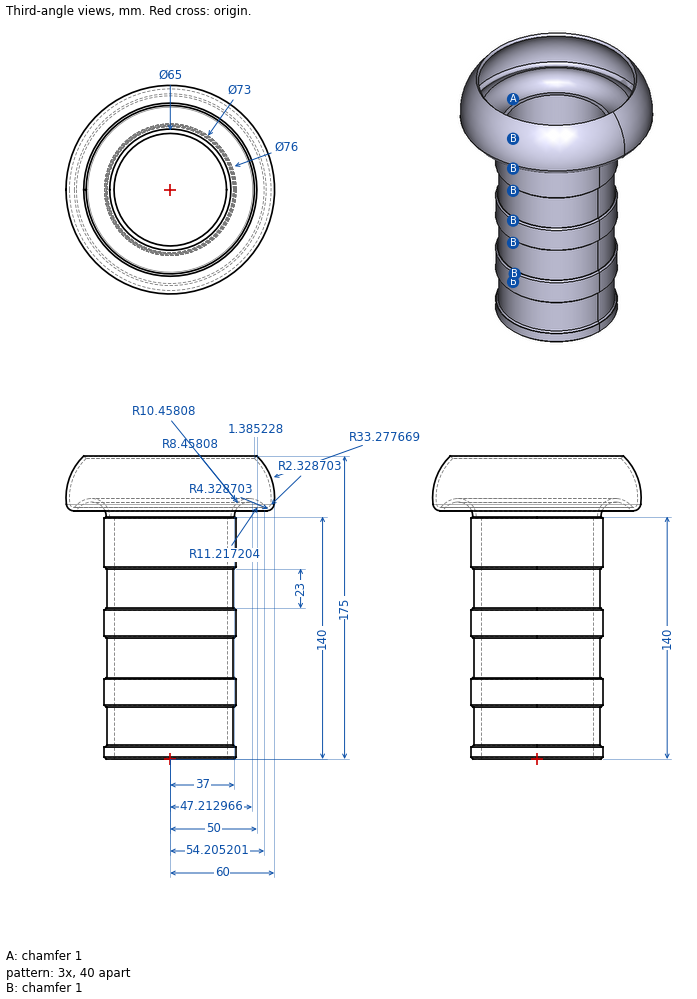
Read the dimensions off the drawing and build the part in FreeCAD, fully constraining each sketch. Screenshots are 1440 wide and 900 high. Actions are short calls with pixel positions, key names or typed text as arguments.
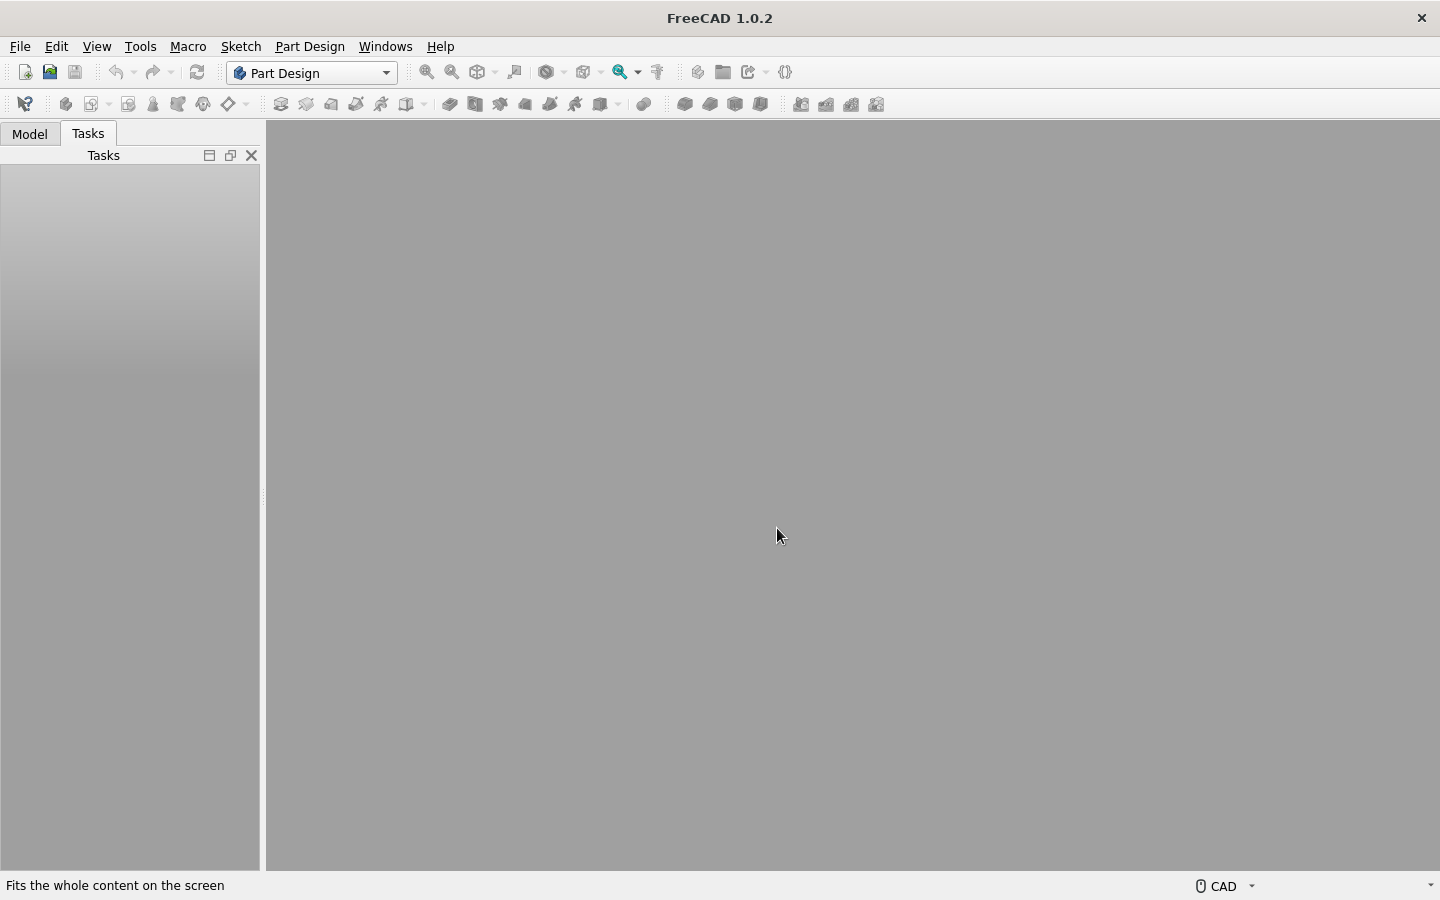
key(ctrl+n)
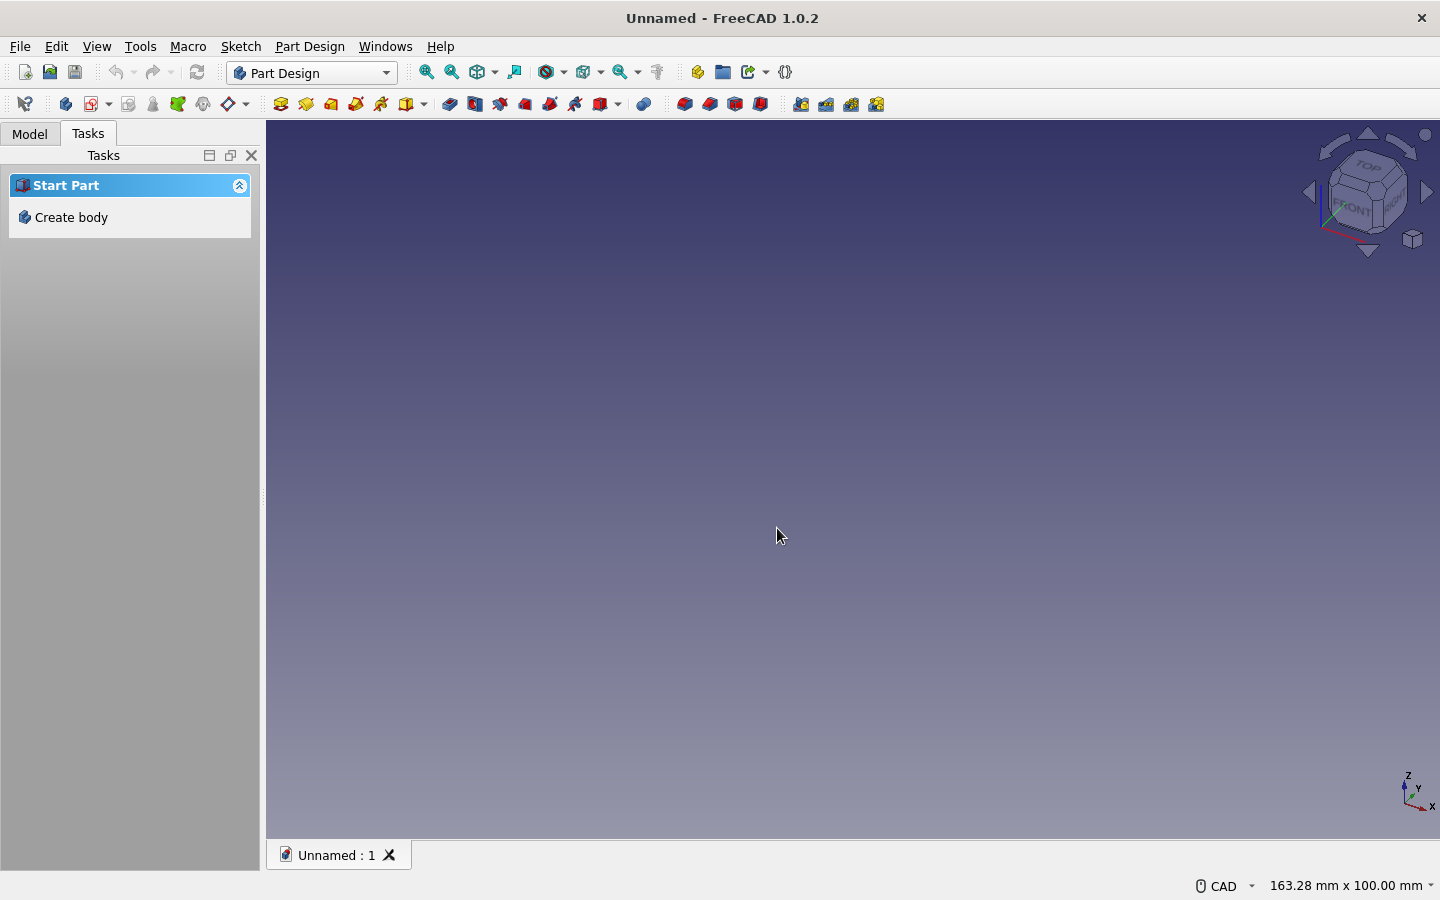
click(90, 104)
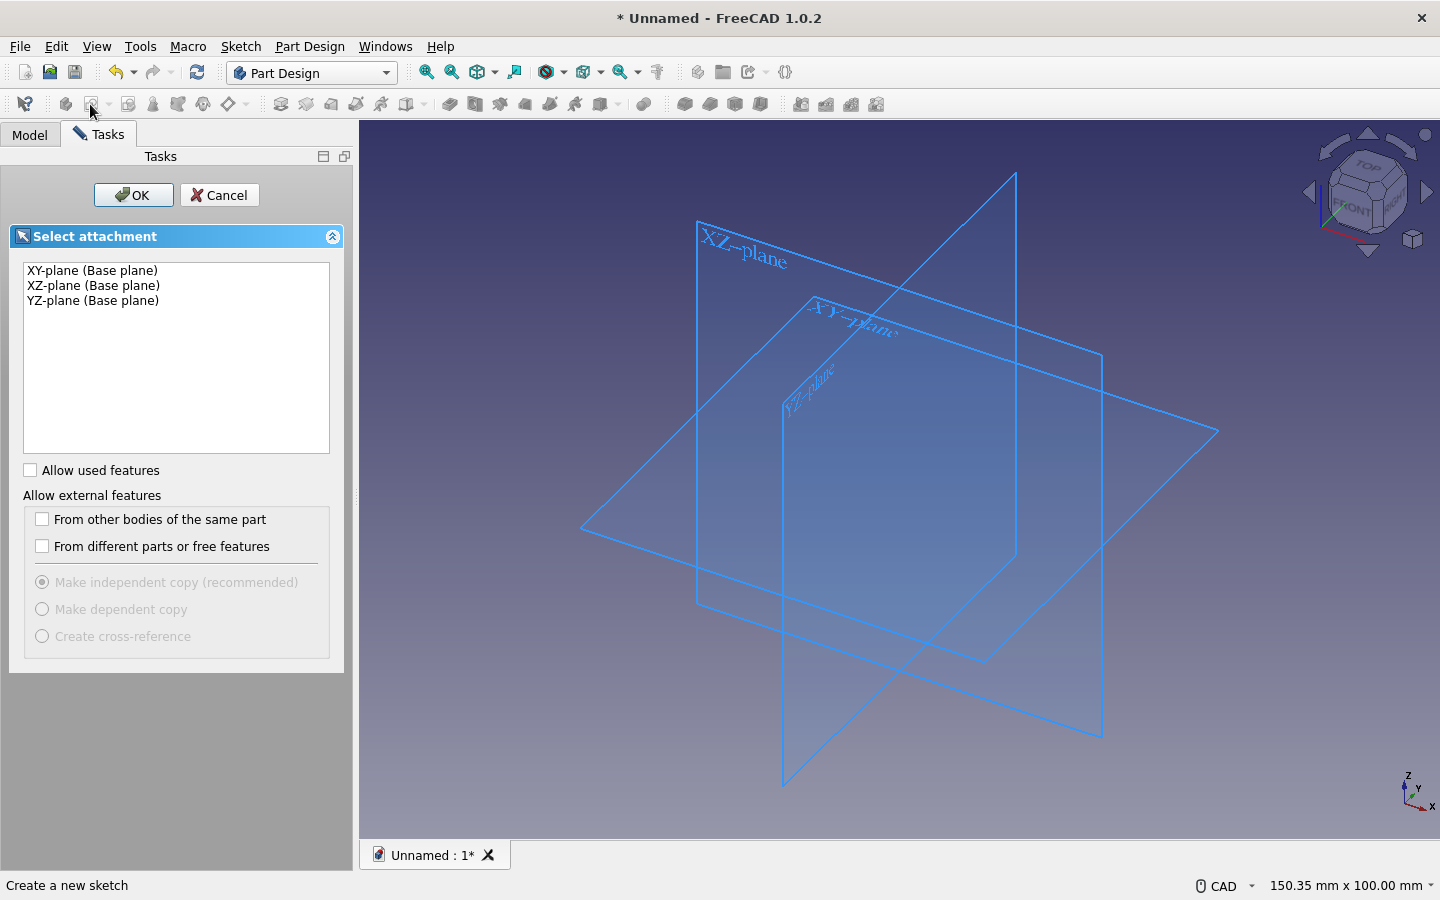
click(84, 270)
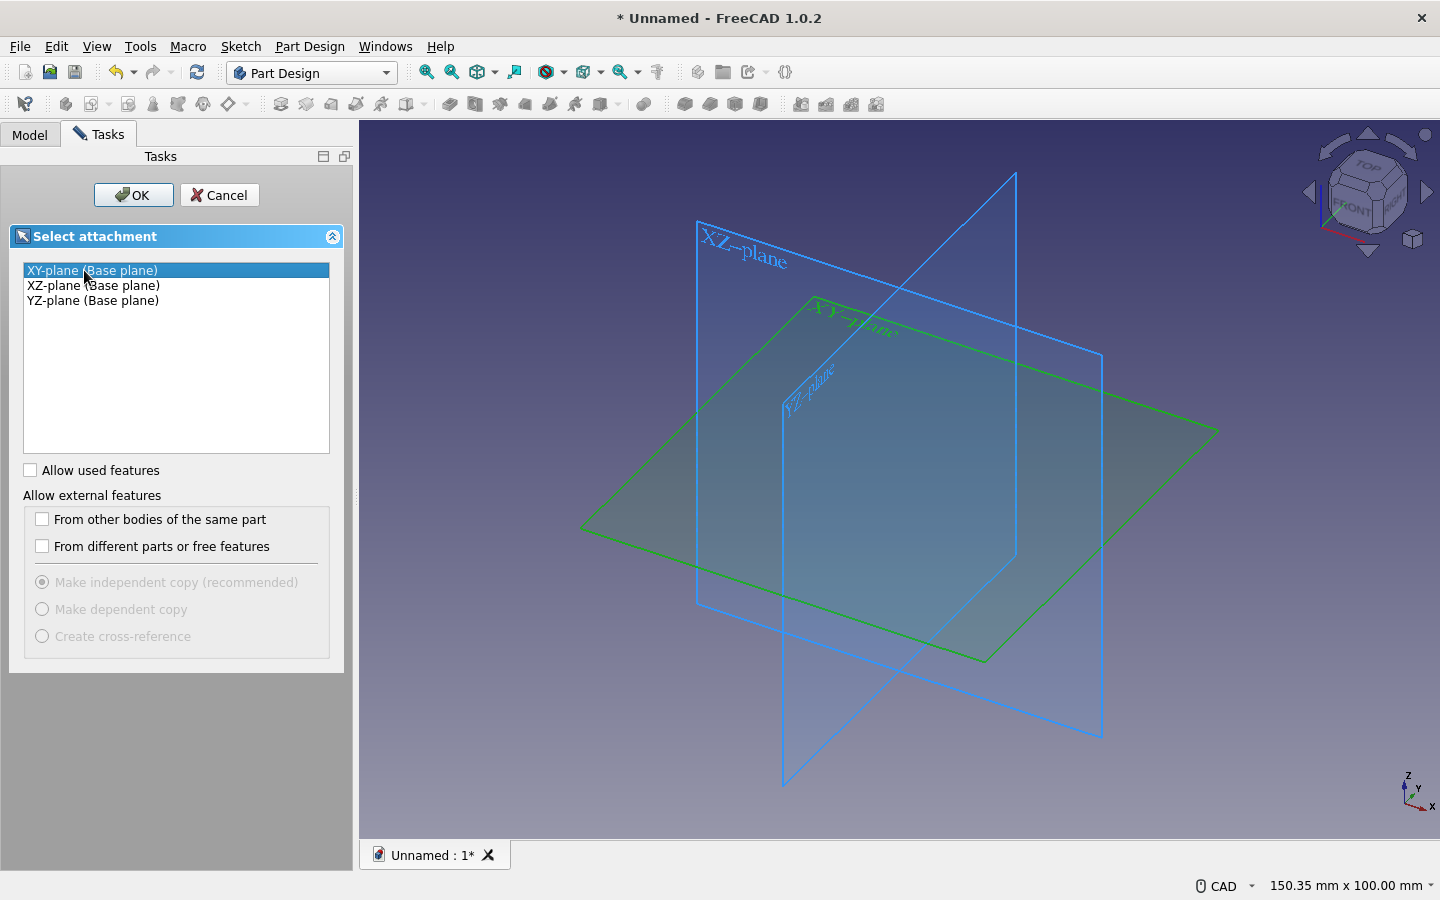
click(134, 195)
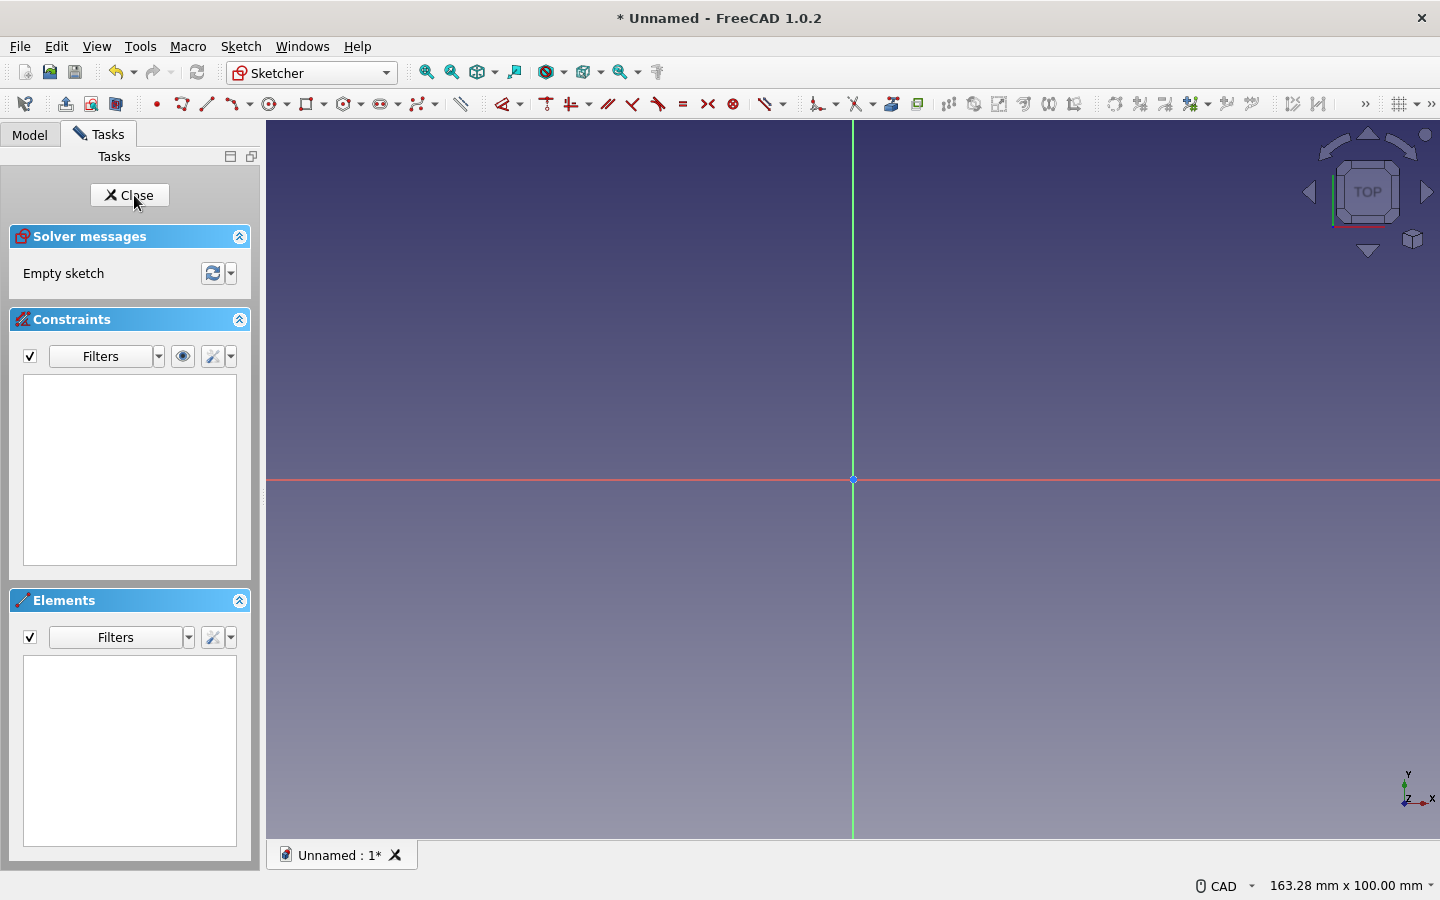
click(268, 104)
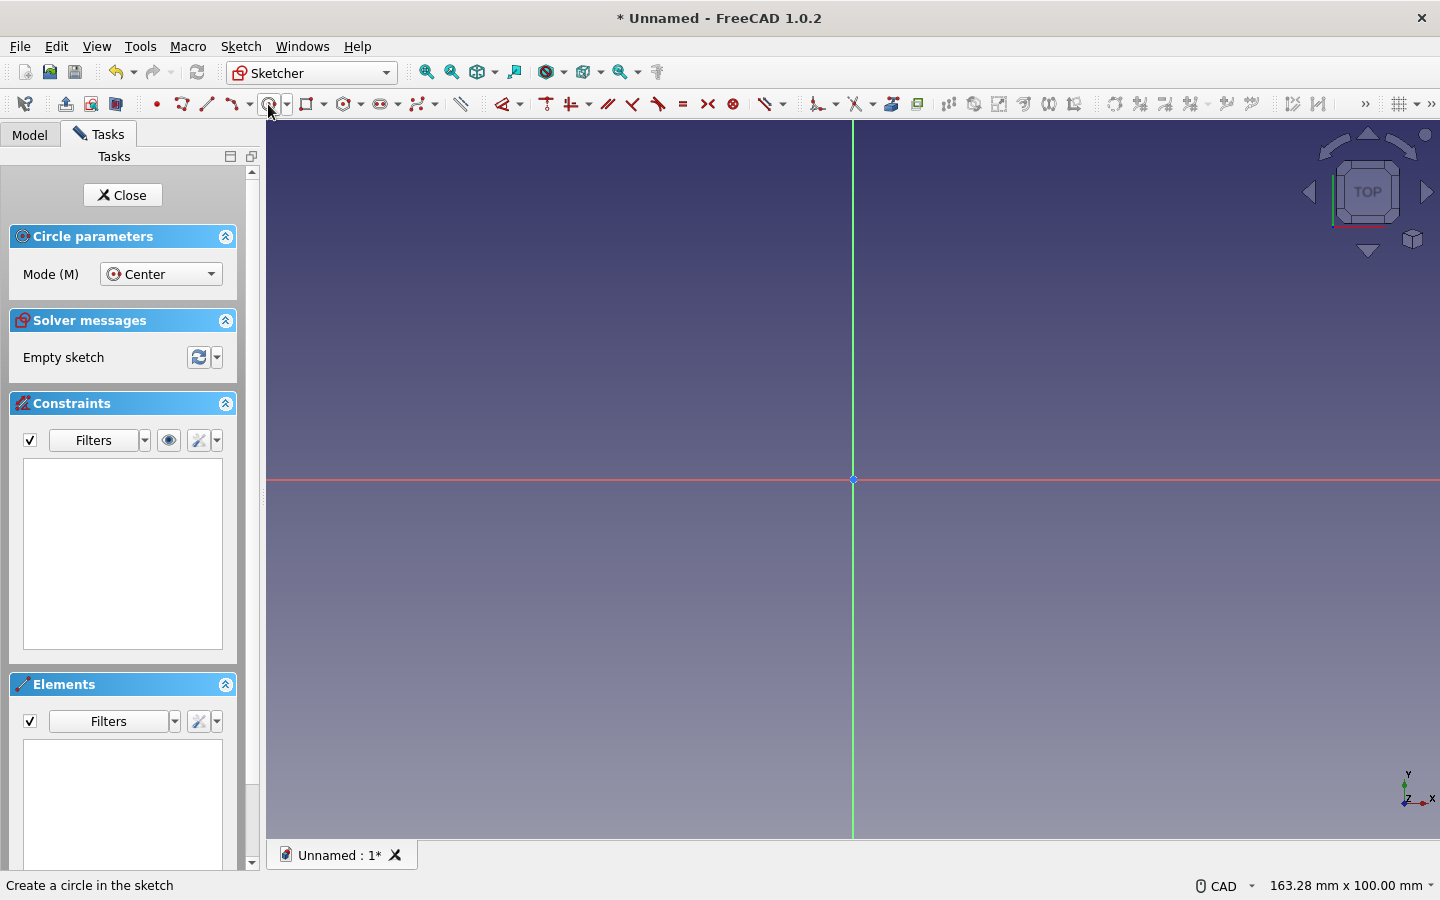
click(853, 480)
move(1046, 286)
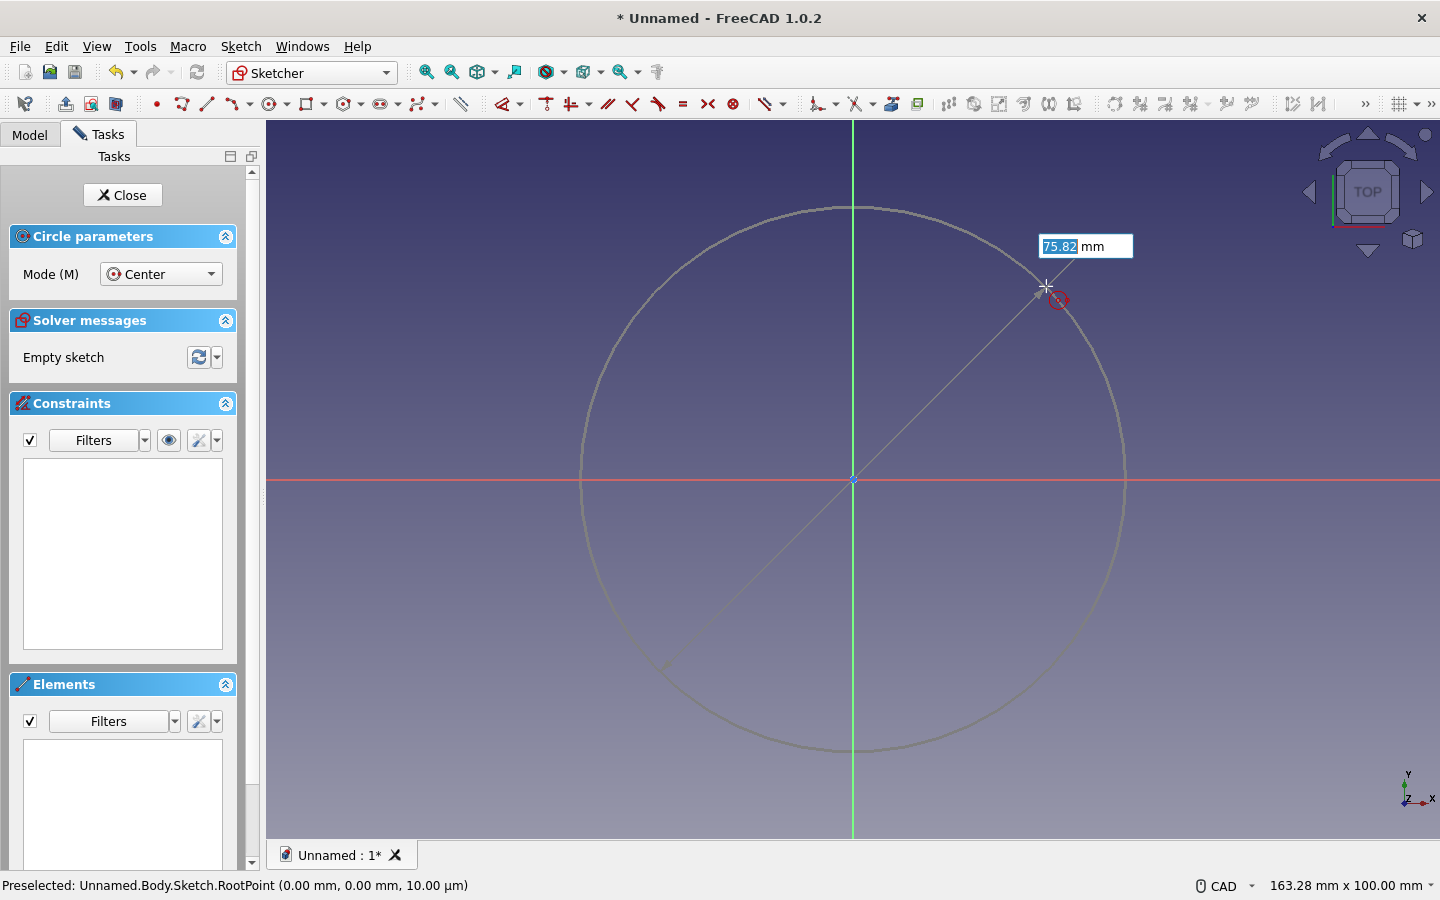
text(76)
key(Return)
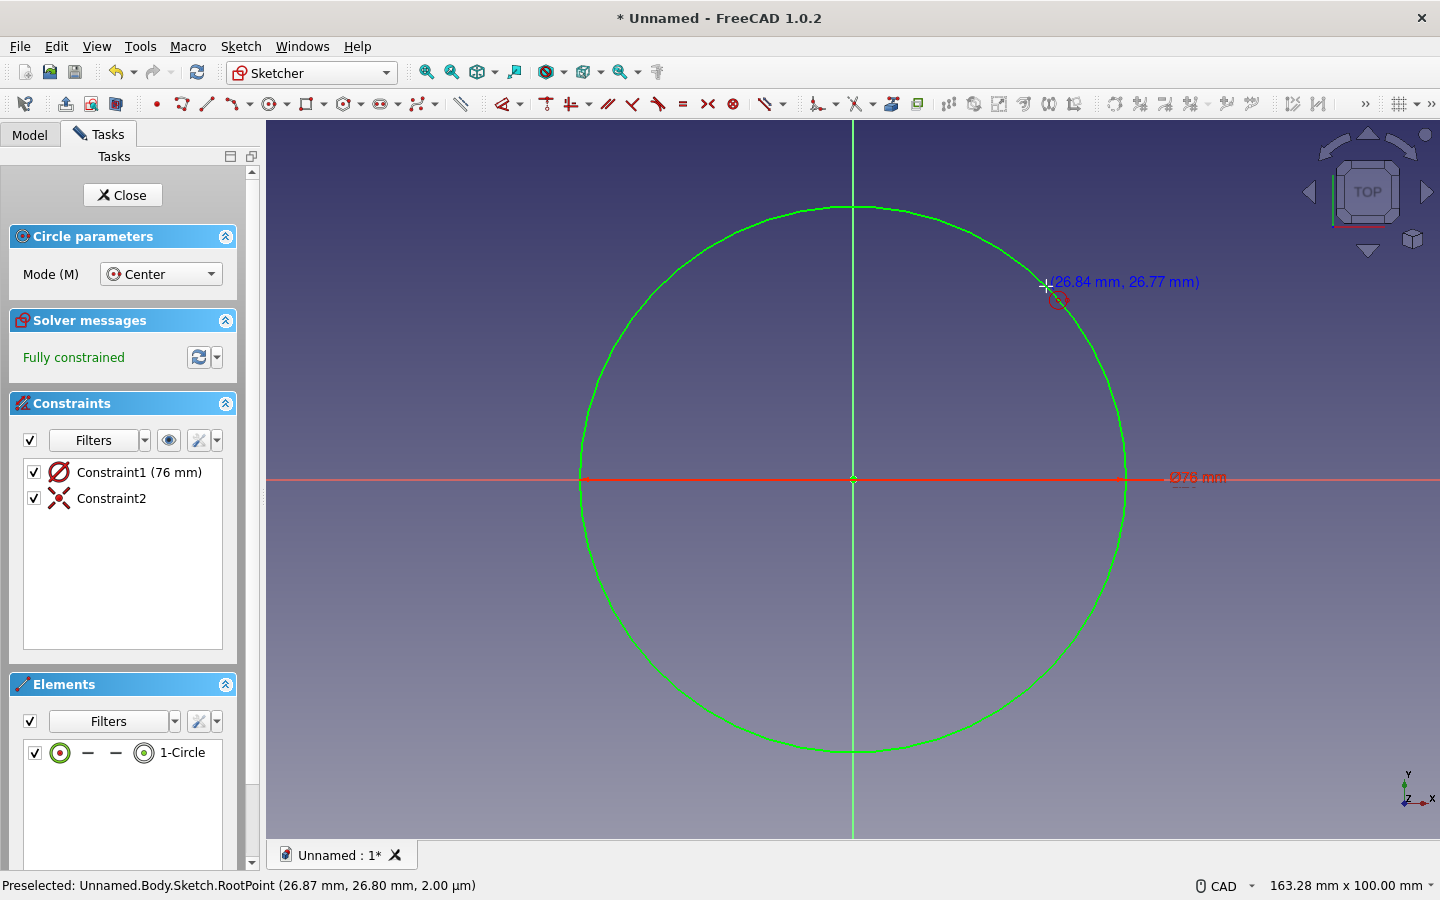
click(853, 480)
move(1018, 314)